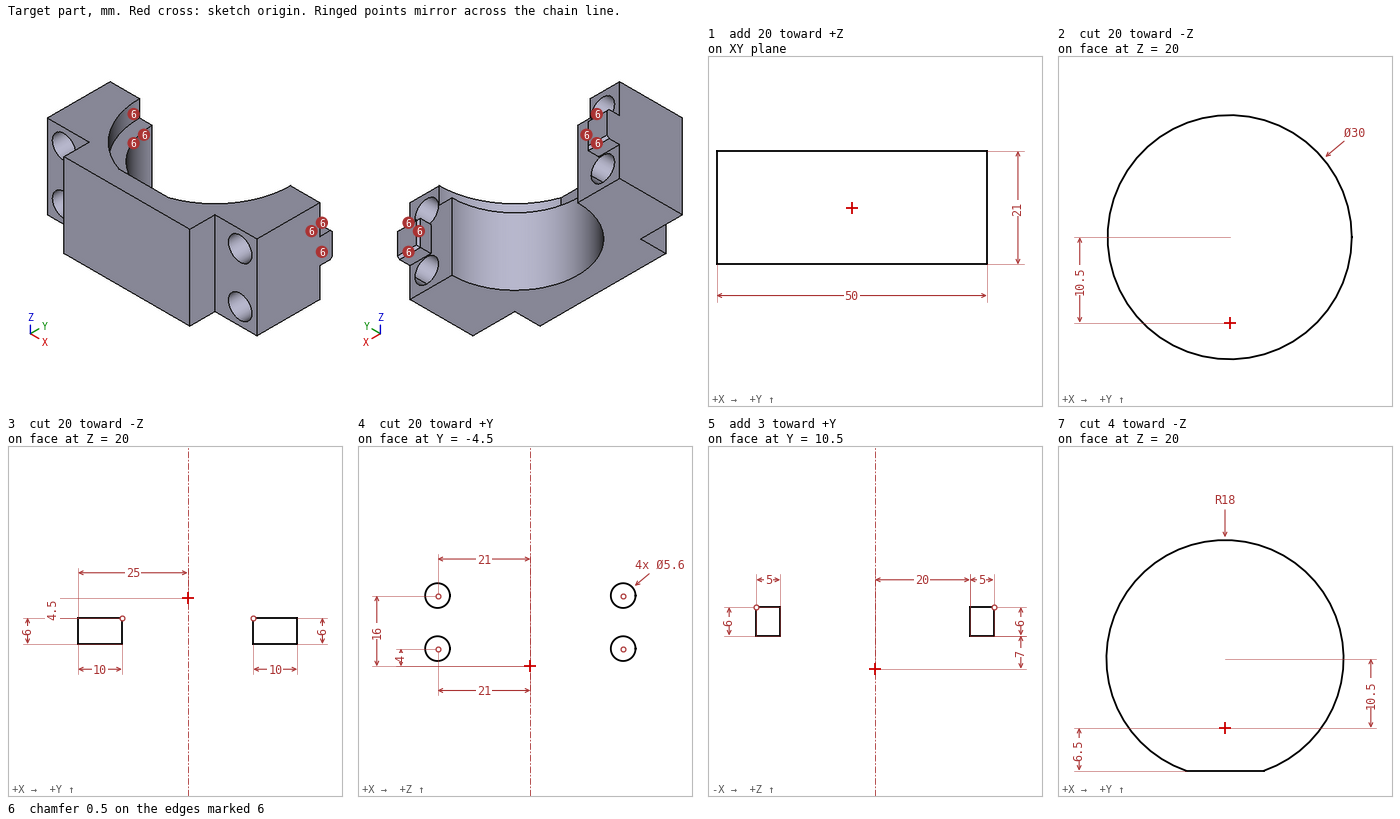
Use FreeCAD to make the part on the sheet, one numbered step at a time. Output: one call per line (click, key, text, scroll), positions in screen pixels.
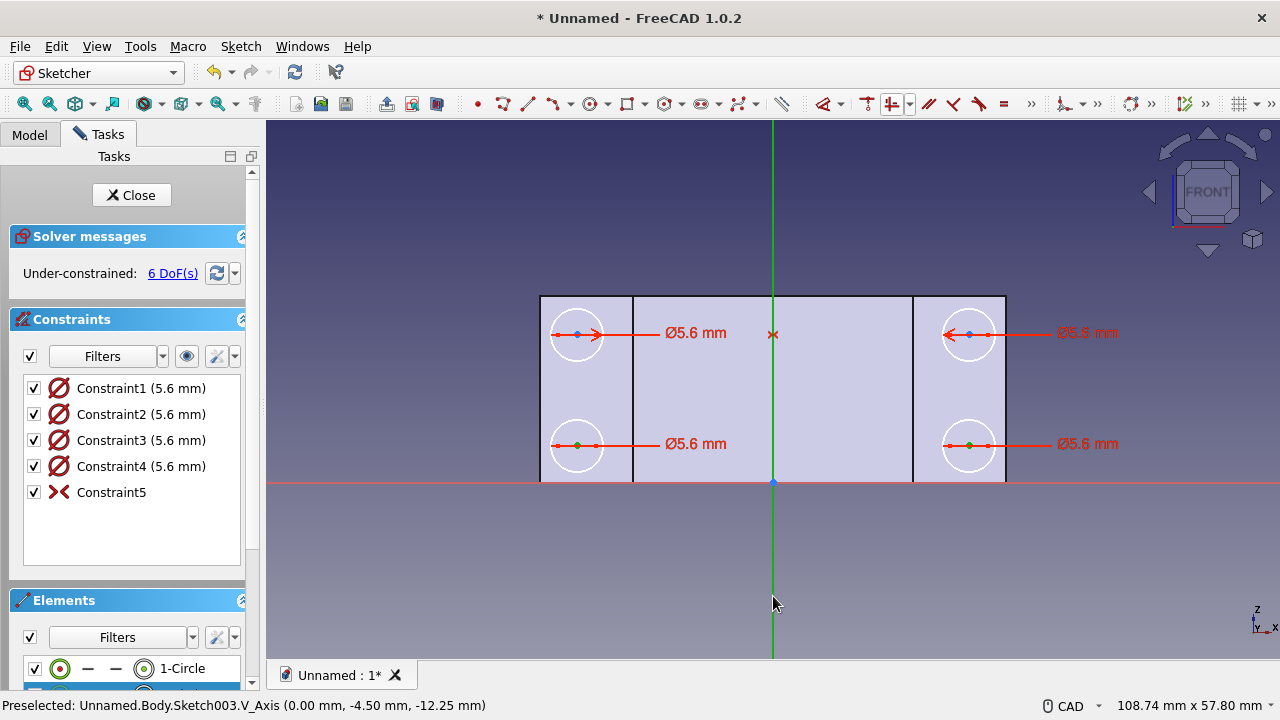
key(s)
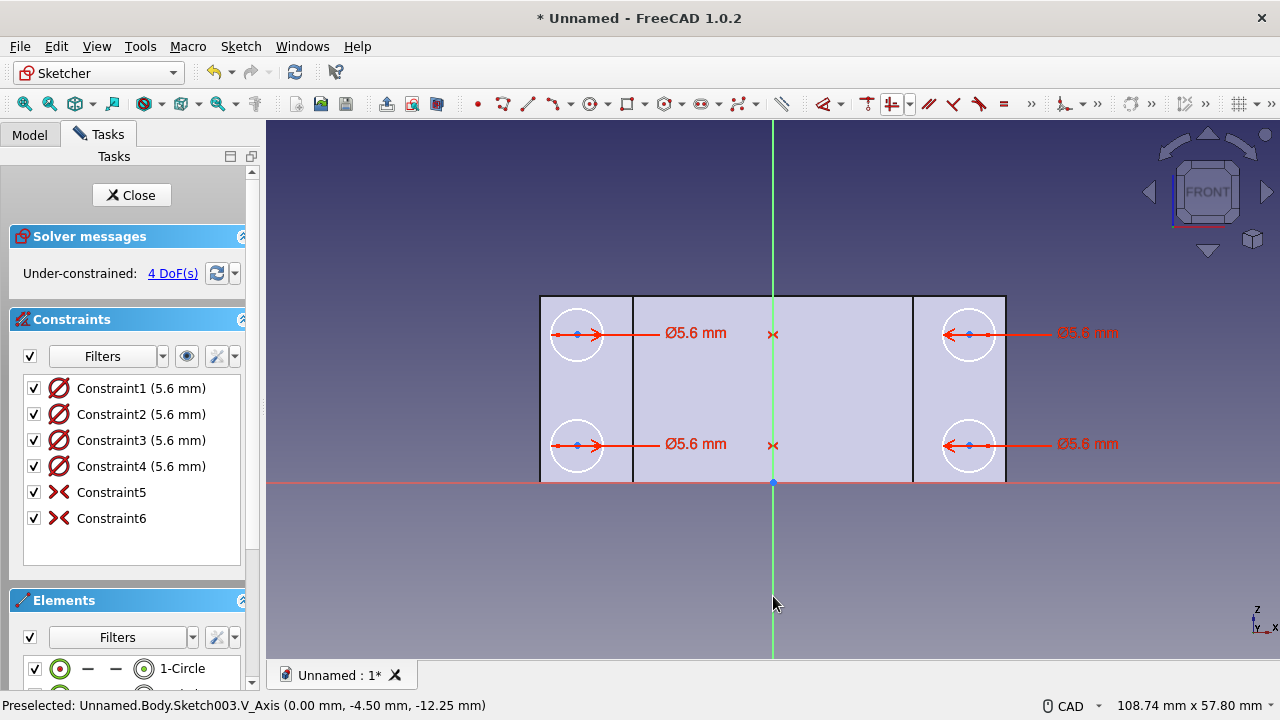
key(d)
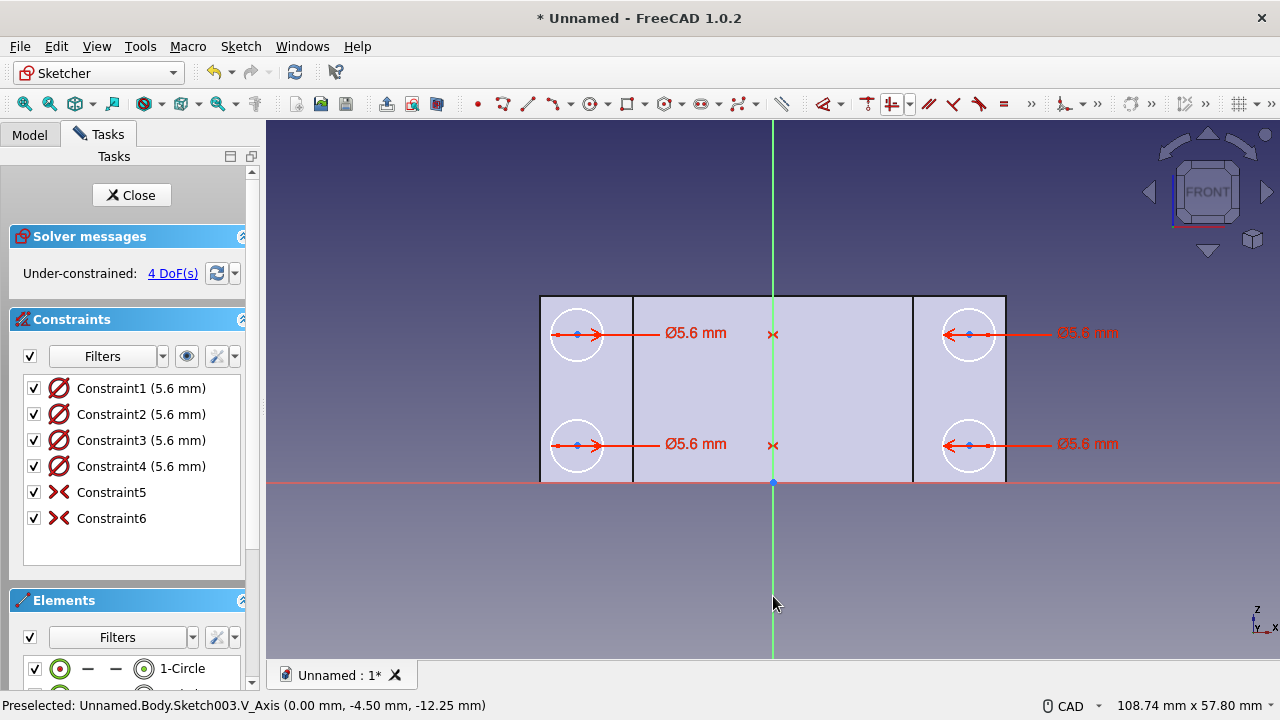
click(577, 446)
click(807, 464)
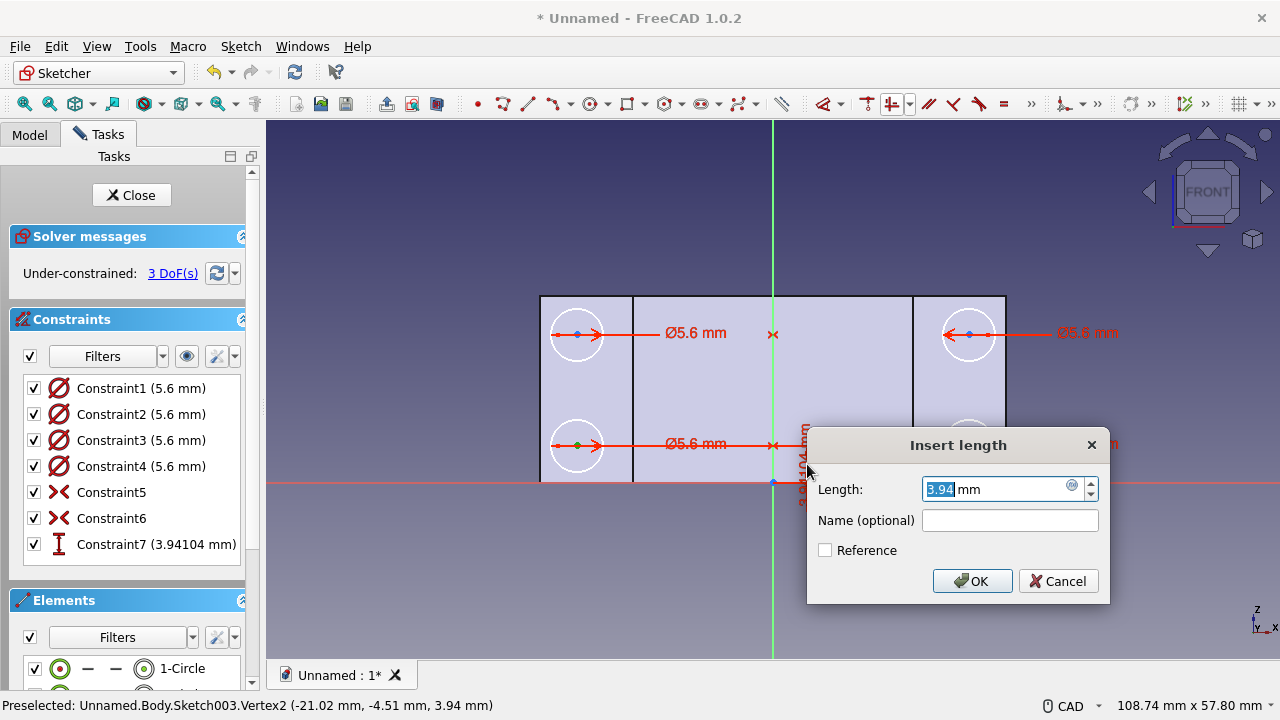
text(4)
key(Return)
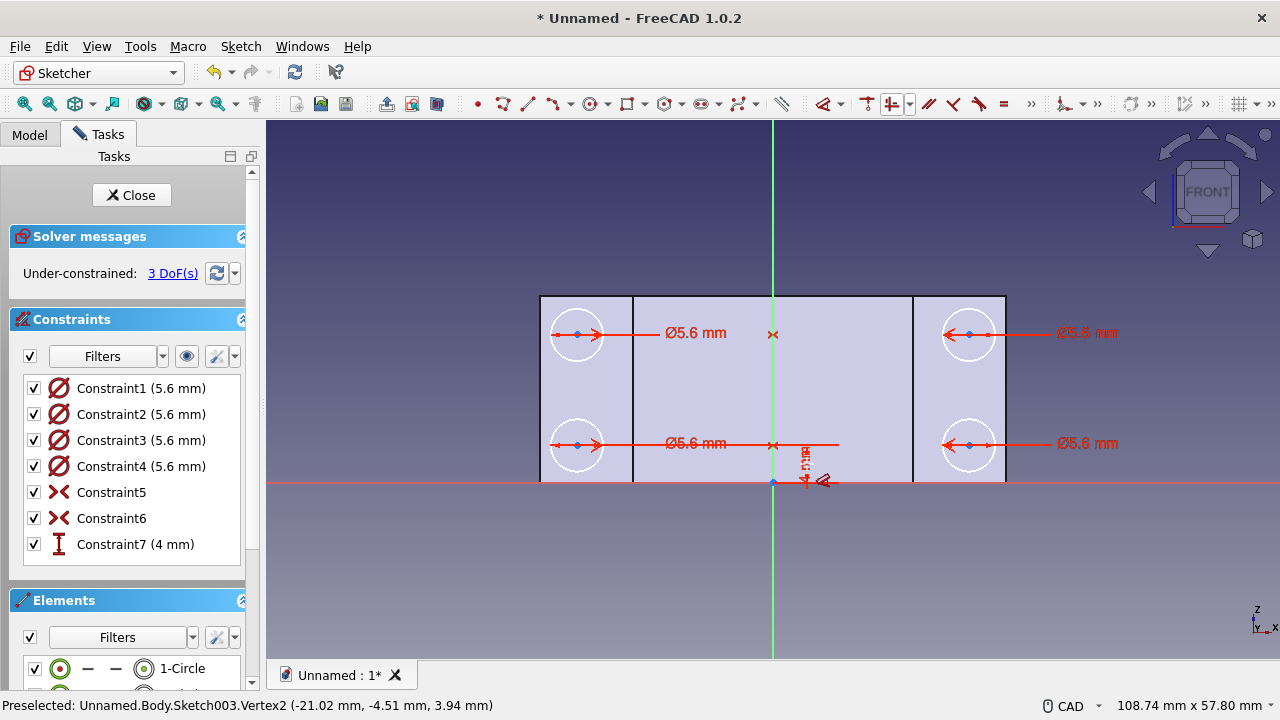
click(577, 335)
click(675, 517)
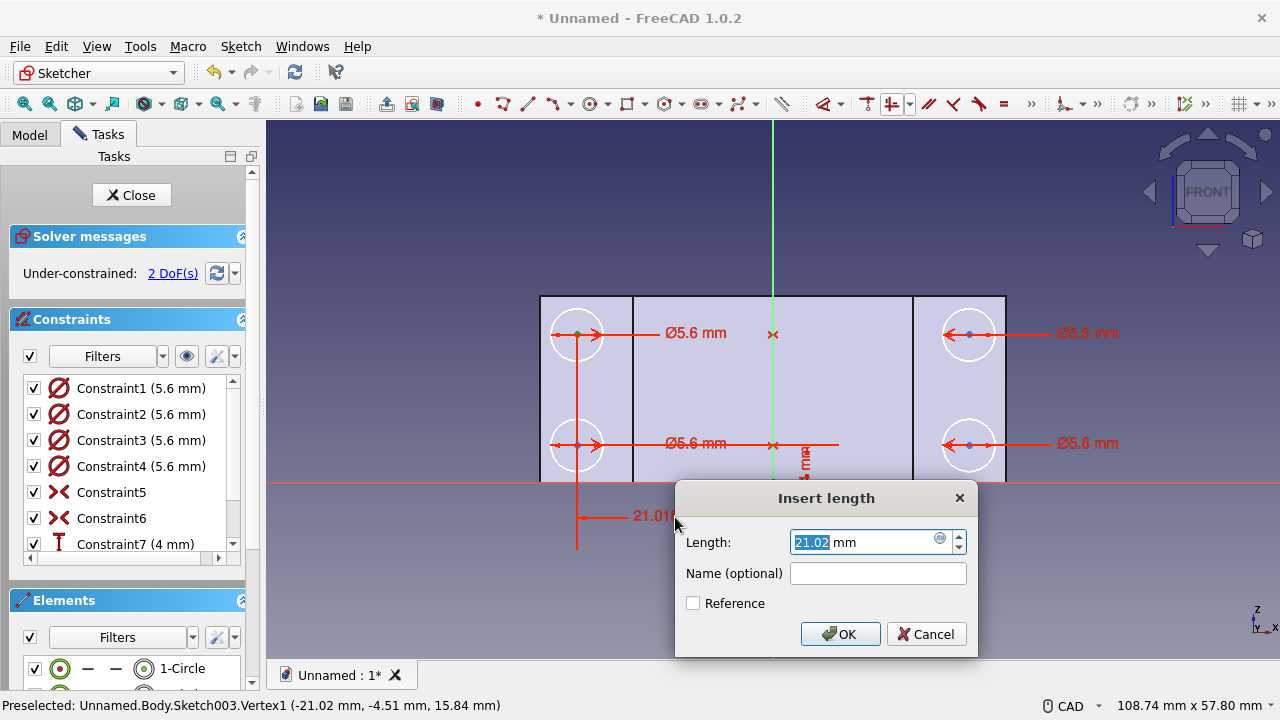
text(21)
key(Return)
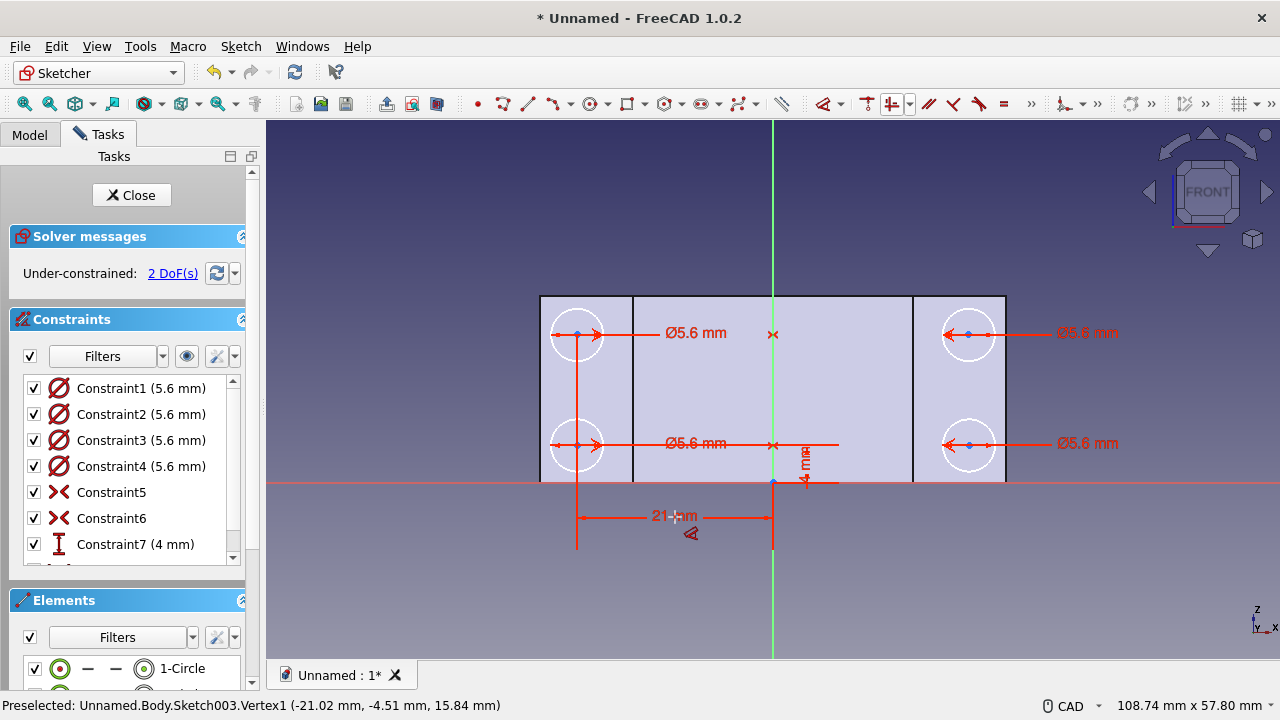
click(577, 335)
click(543, 409)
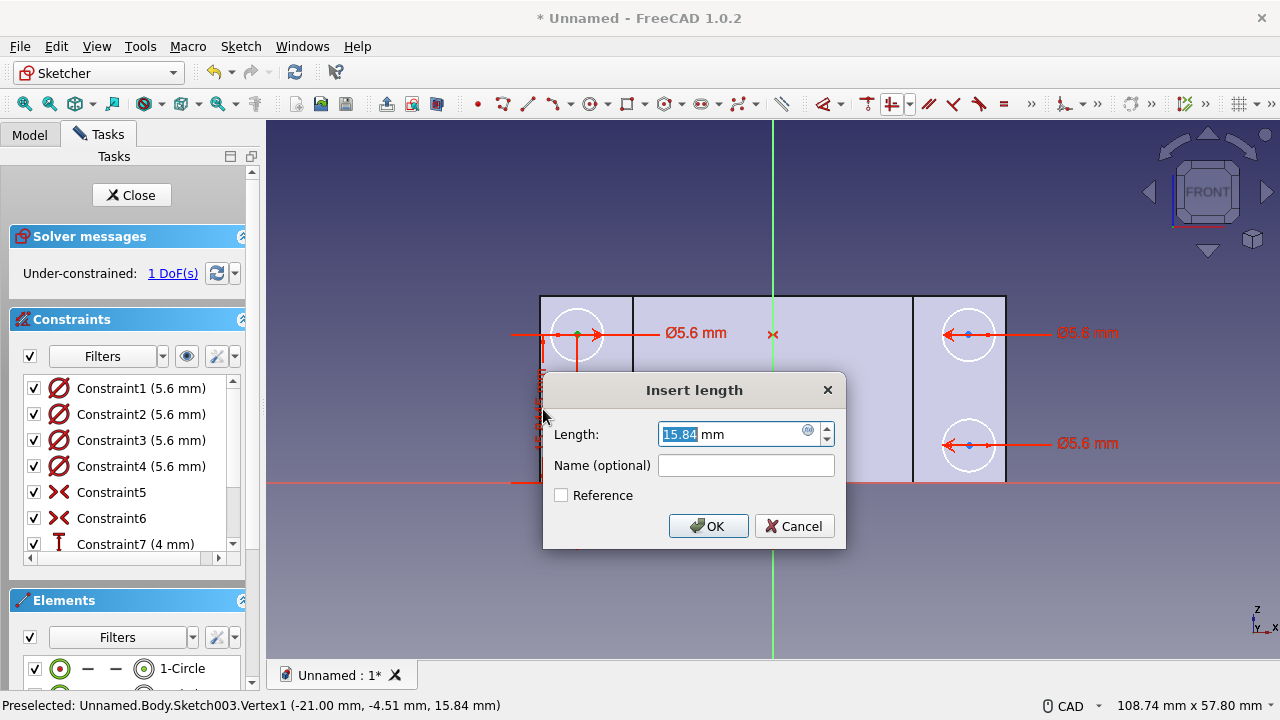
text(16)
key(Return)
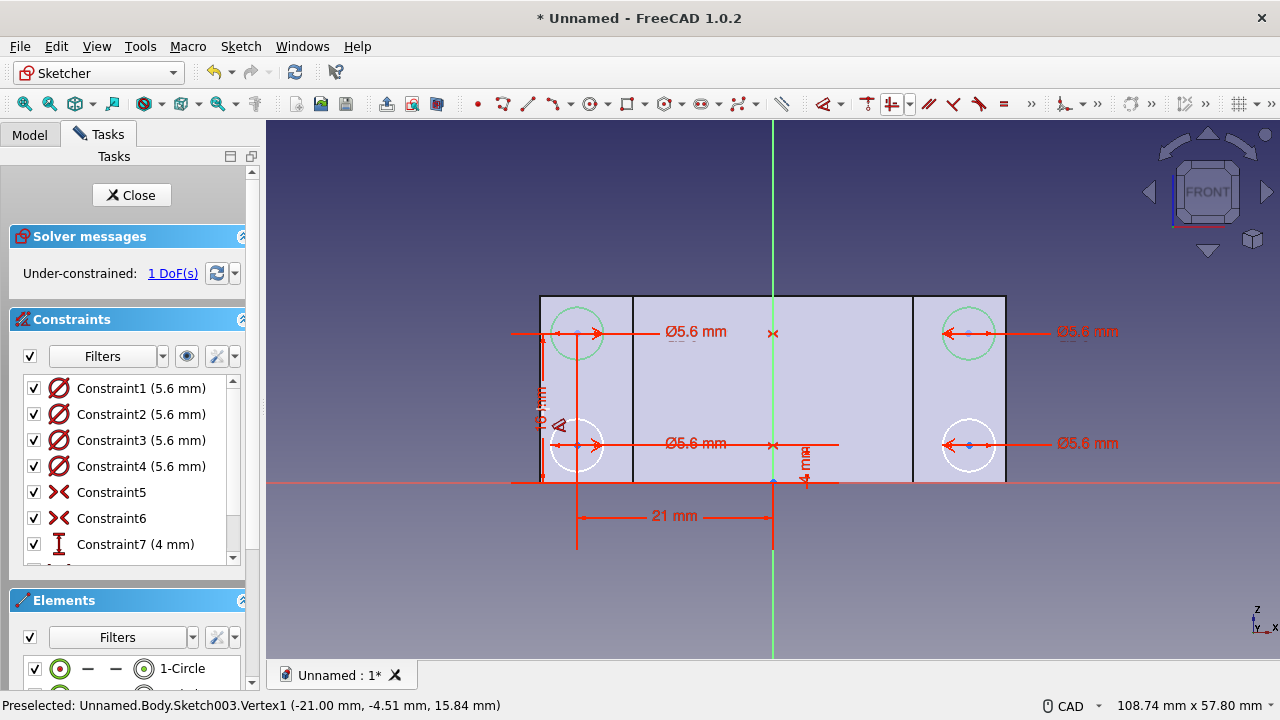
click(577, 445)
click(675, 411)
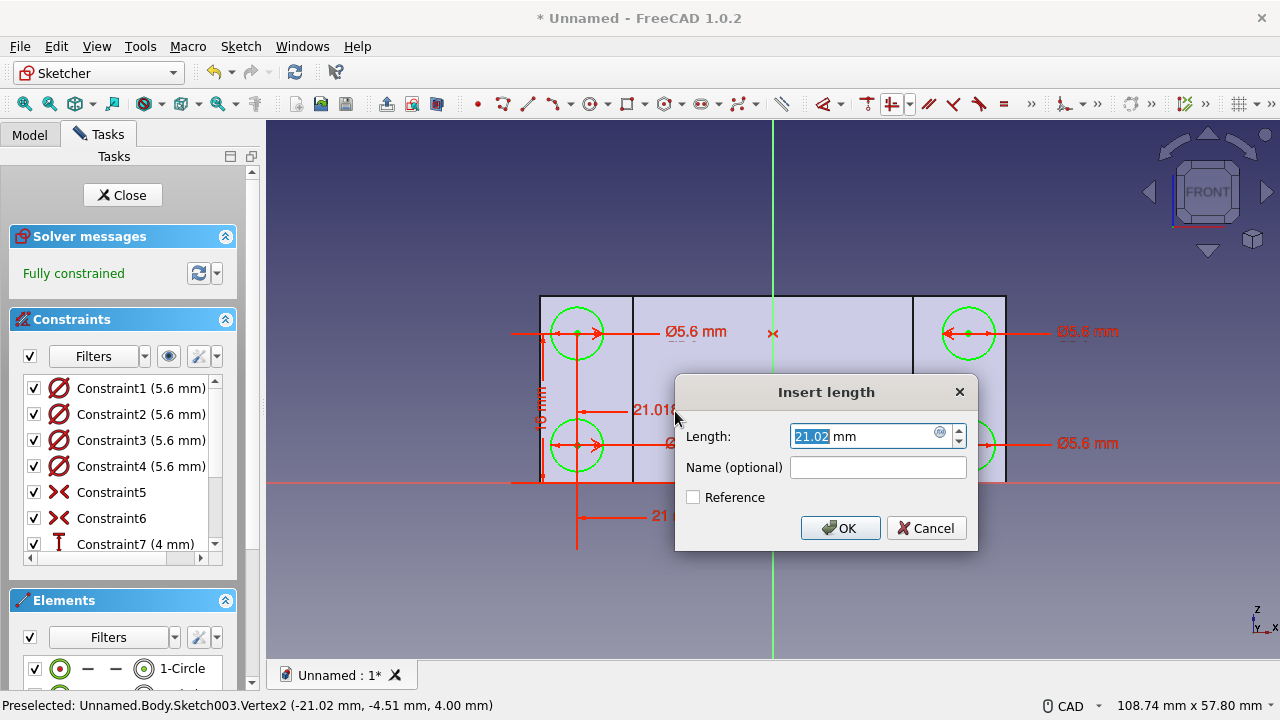
text(21)
key(Return)
key(Escape)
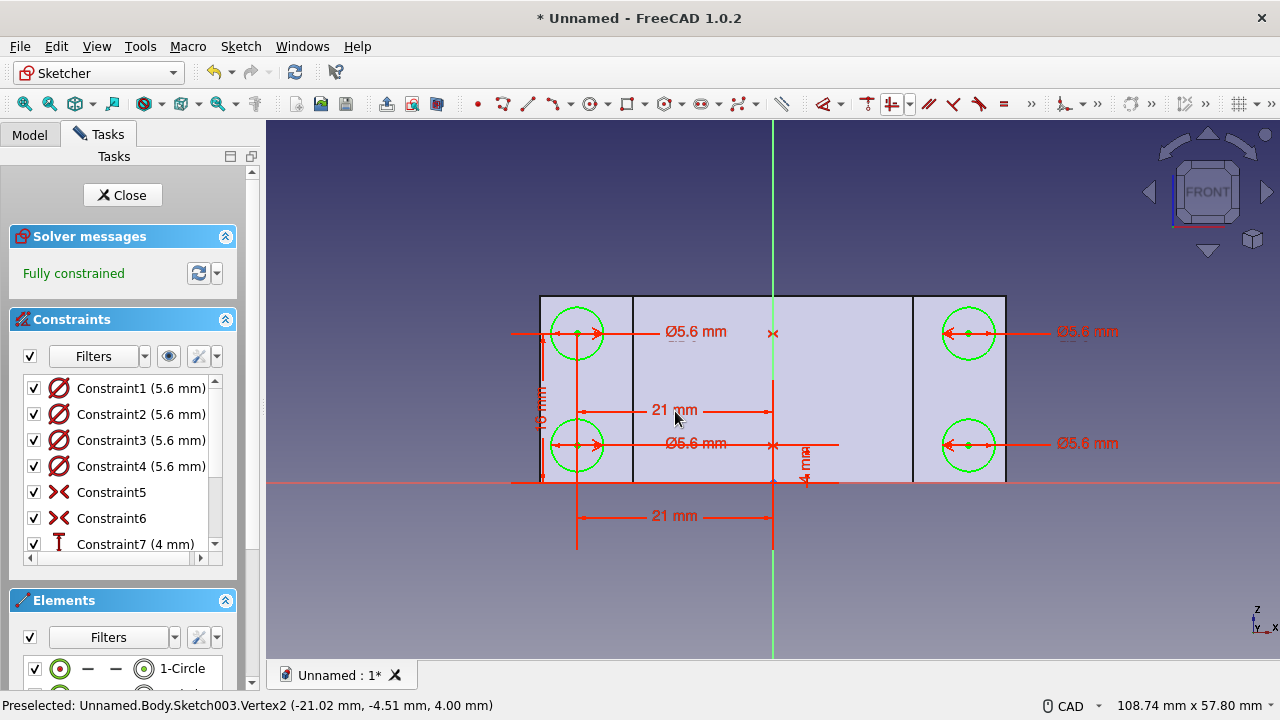
click(123, 195)